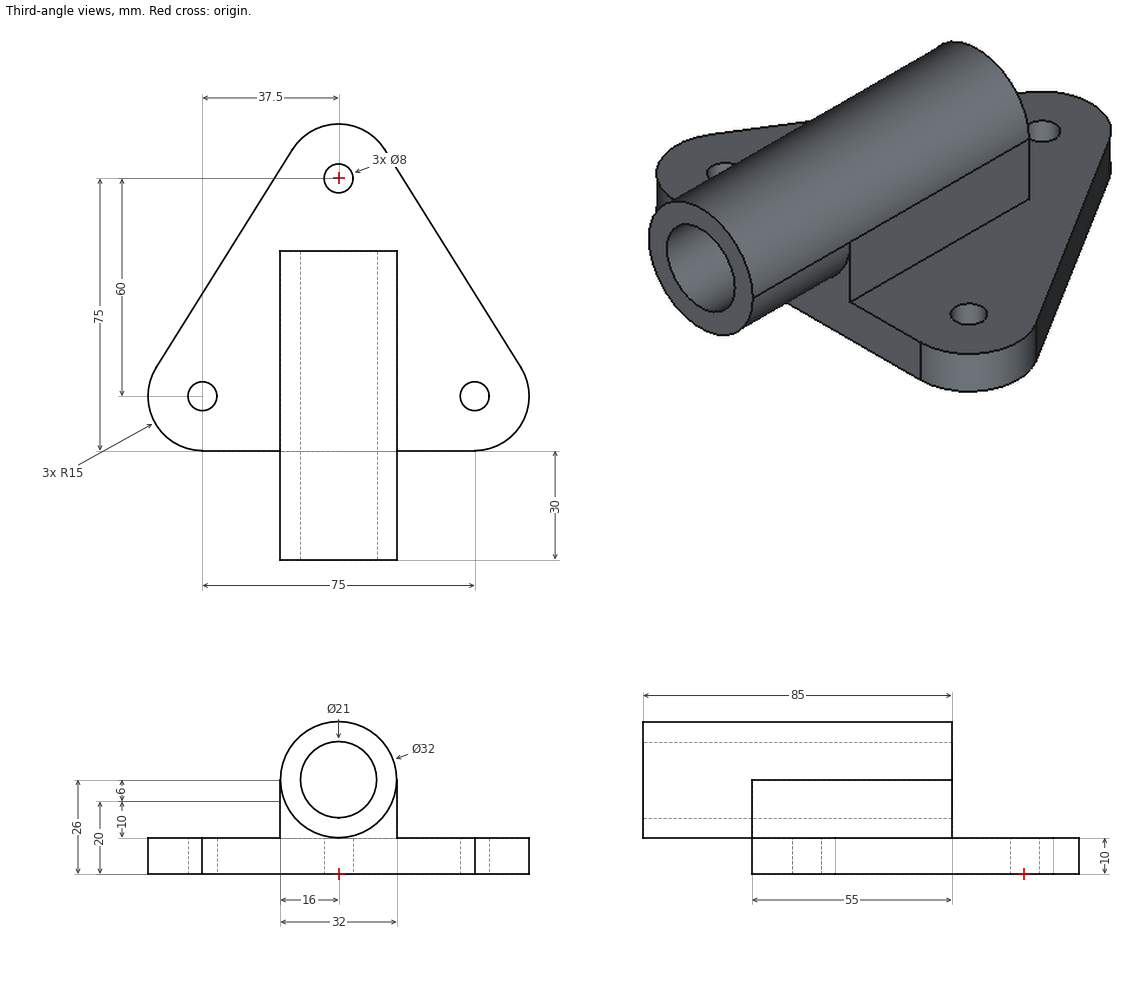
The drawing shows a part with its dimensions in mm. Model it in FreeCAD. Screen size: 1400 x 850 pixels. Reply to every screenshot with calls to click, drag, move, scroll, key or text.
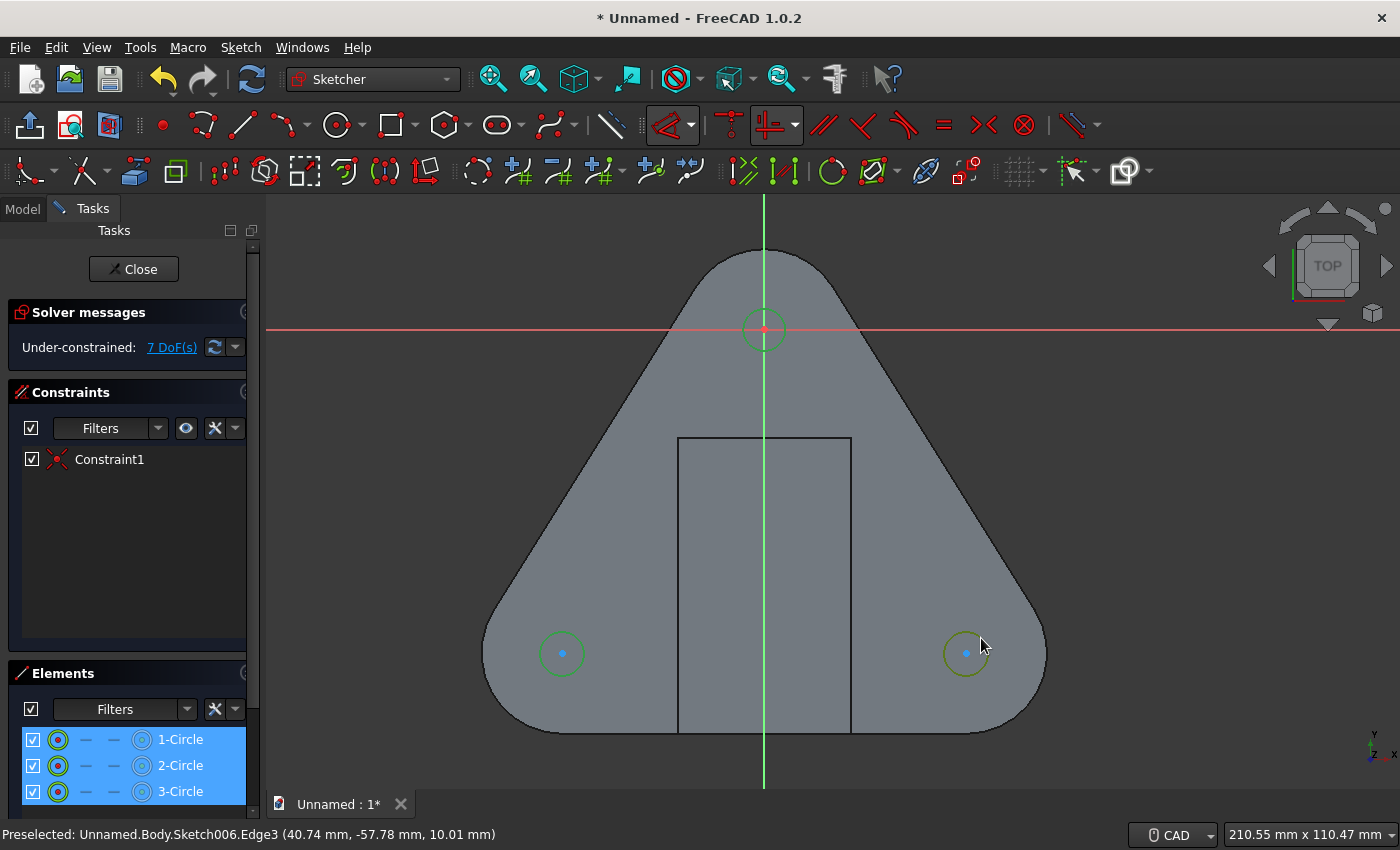
click(944, 126)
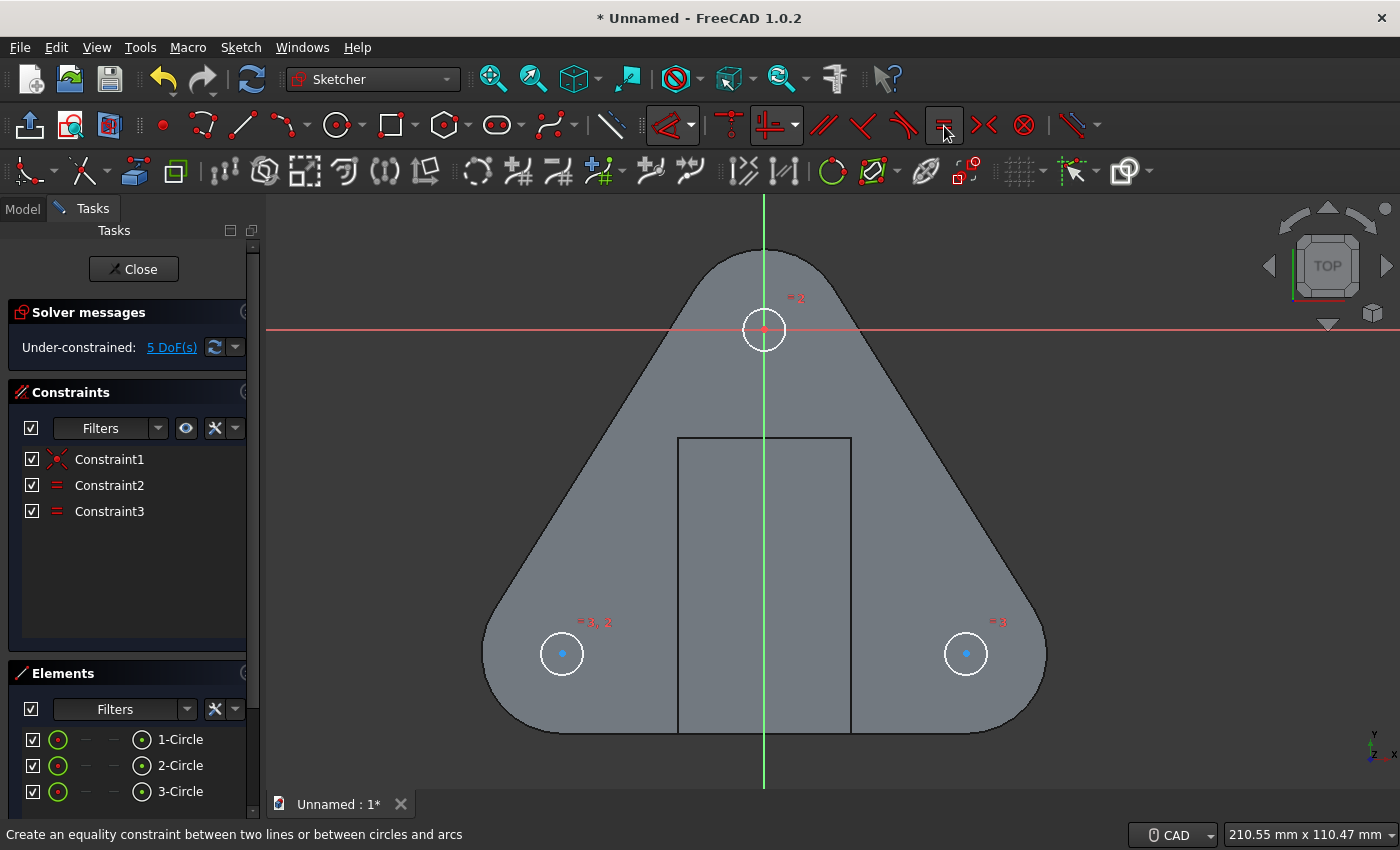
click(562, 654)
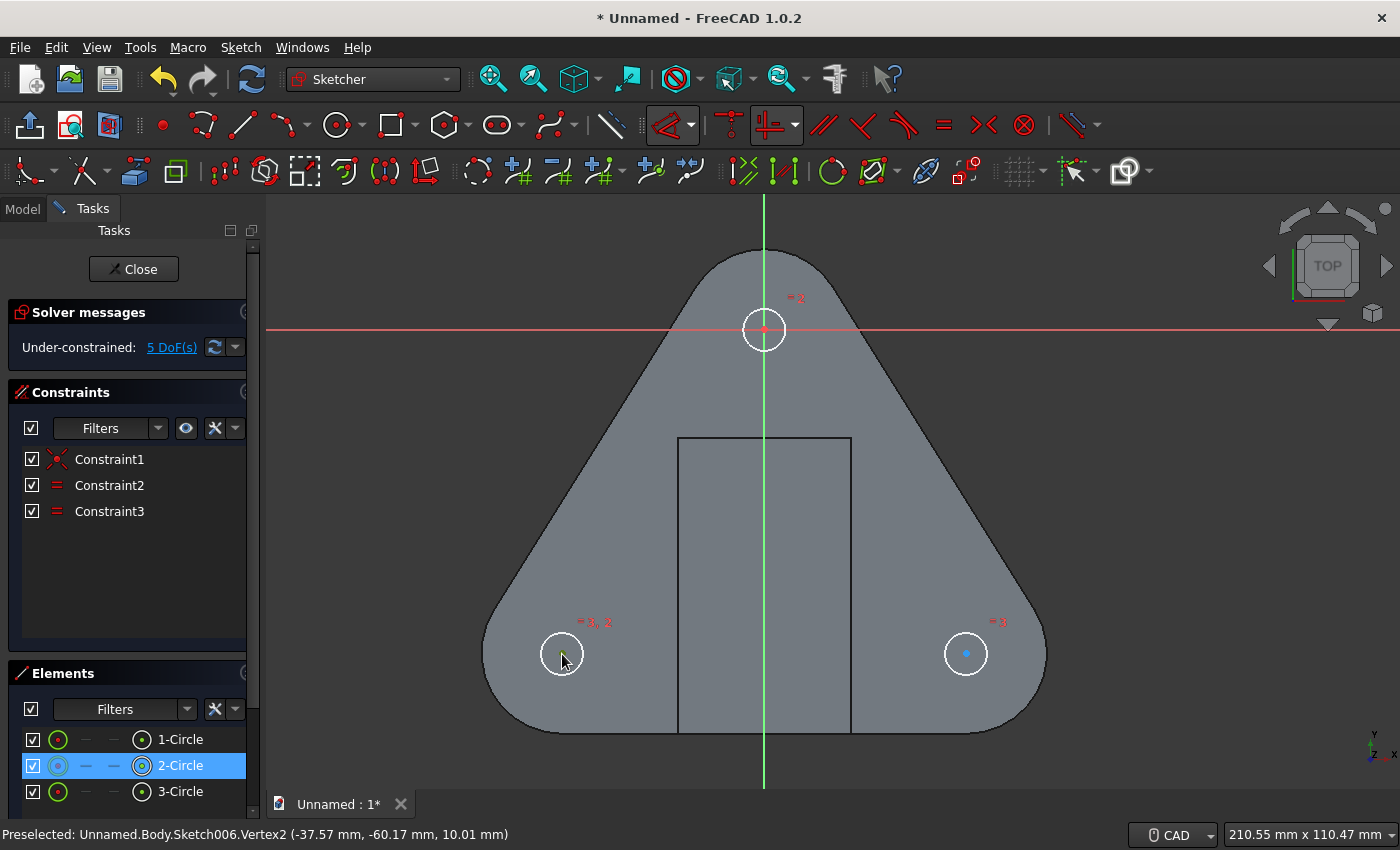
click(966, 654)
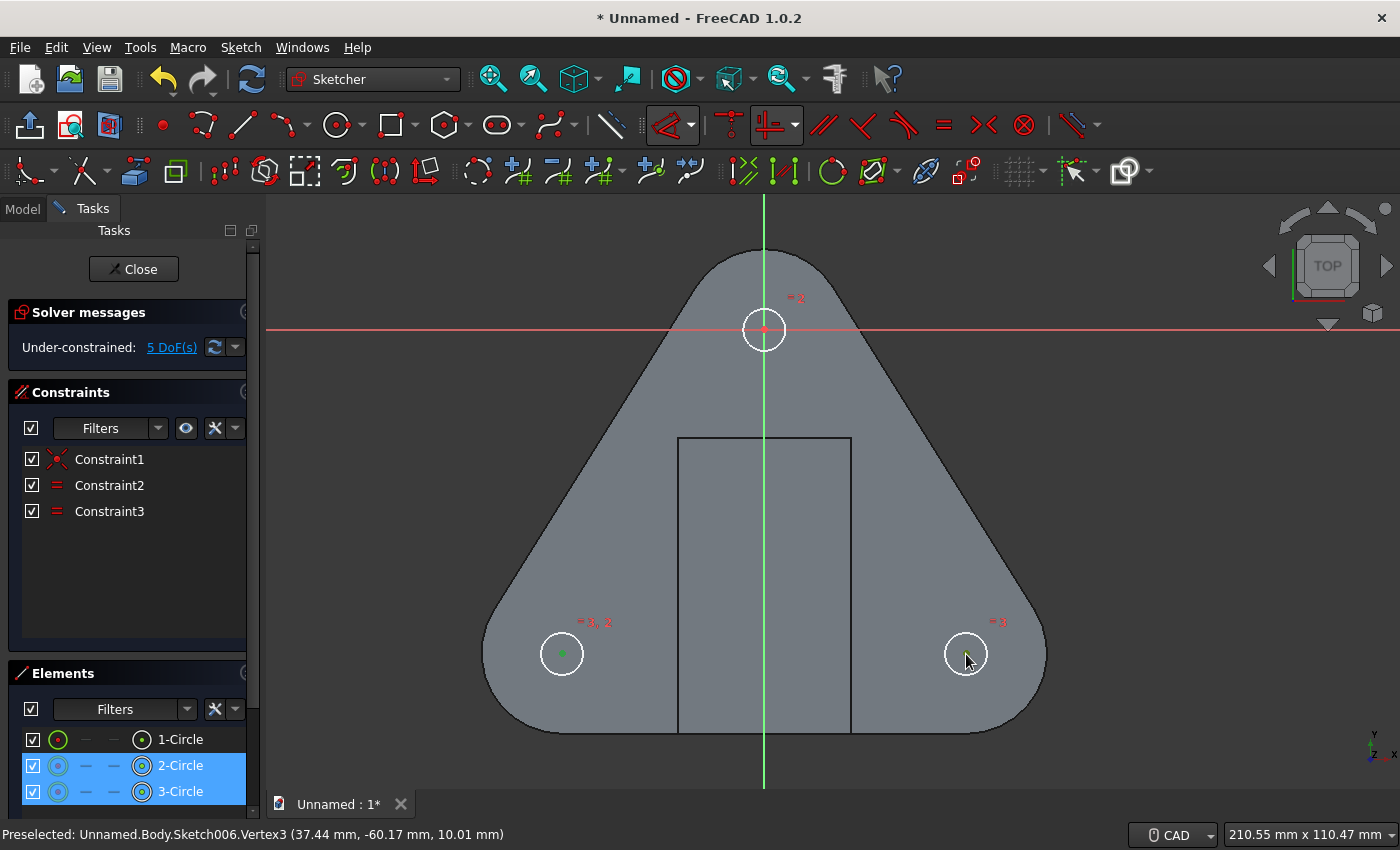
key(h)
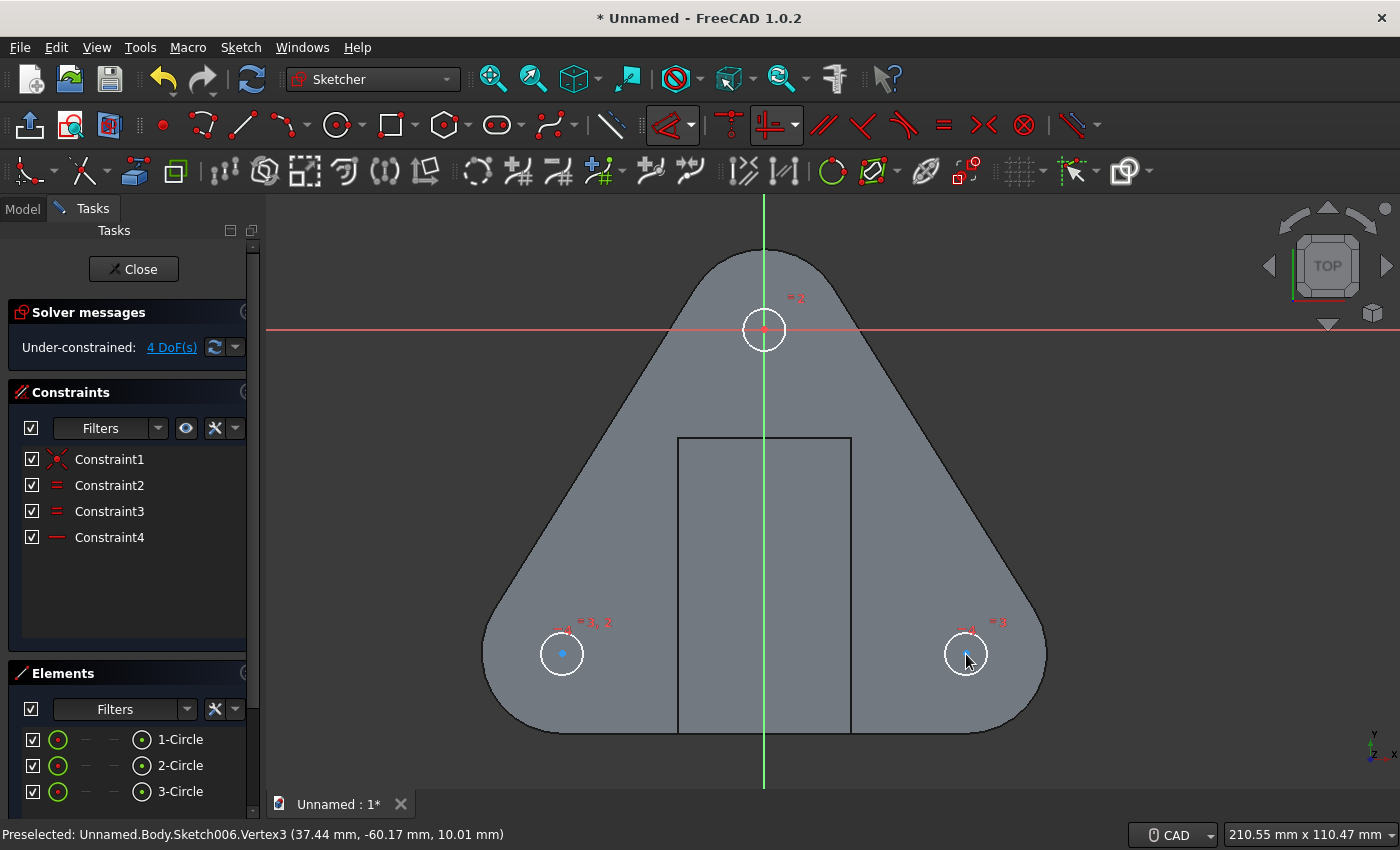
click(779, 315)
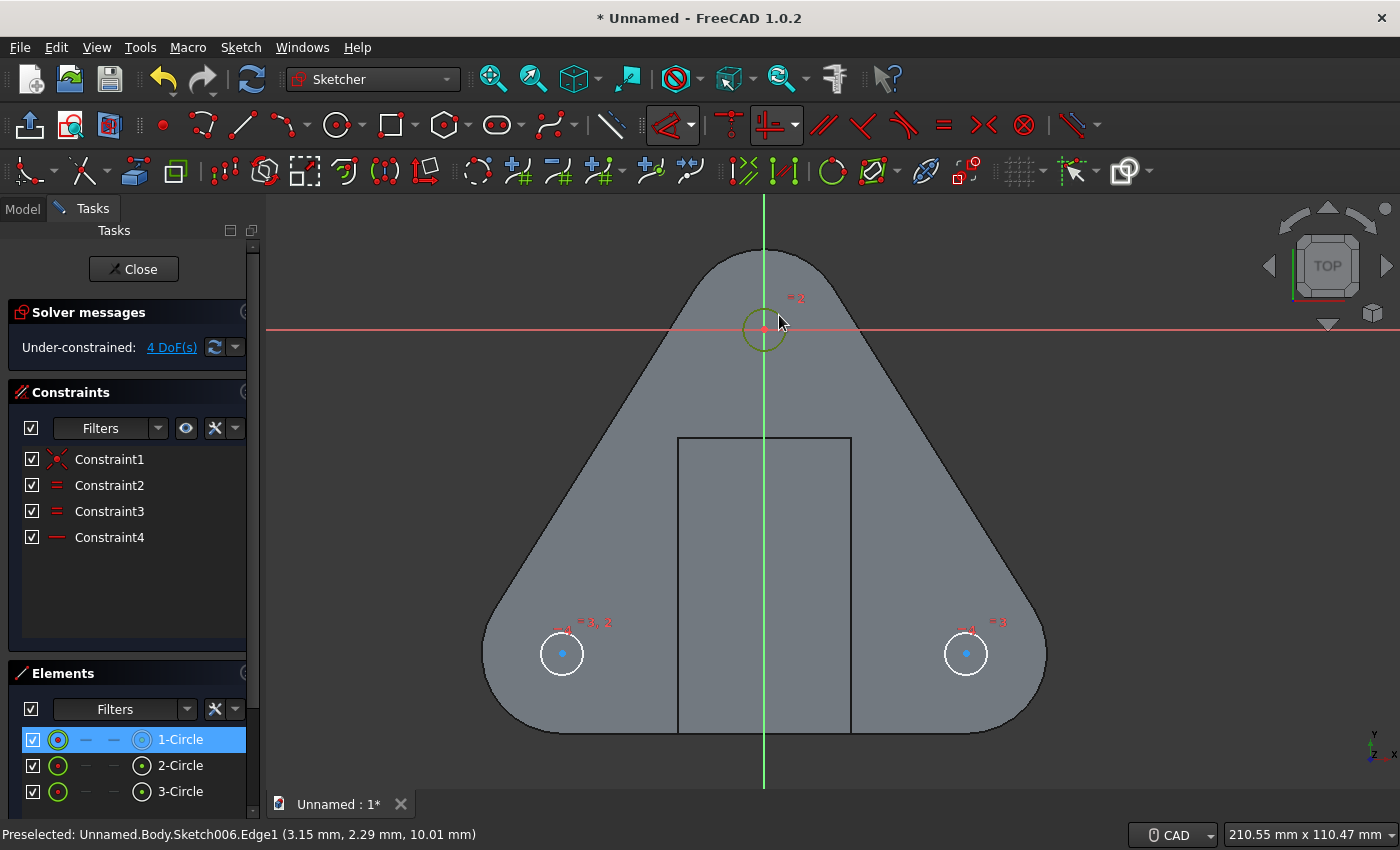
click(694, 126)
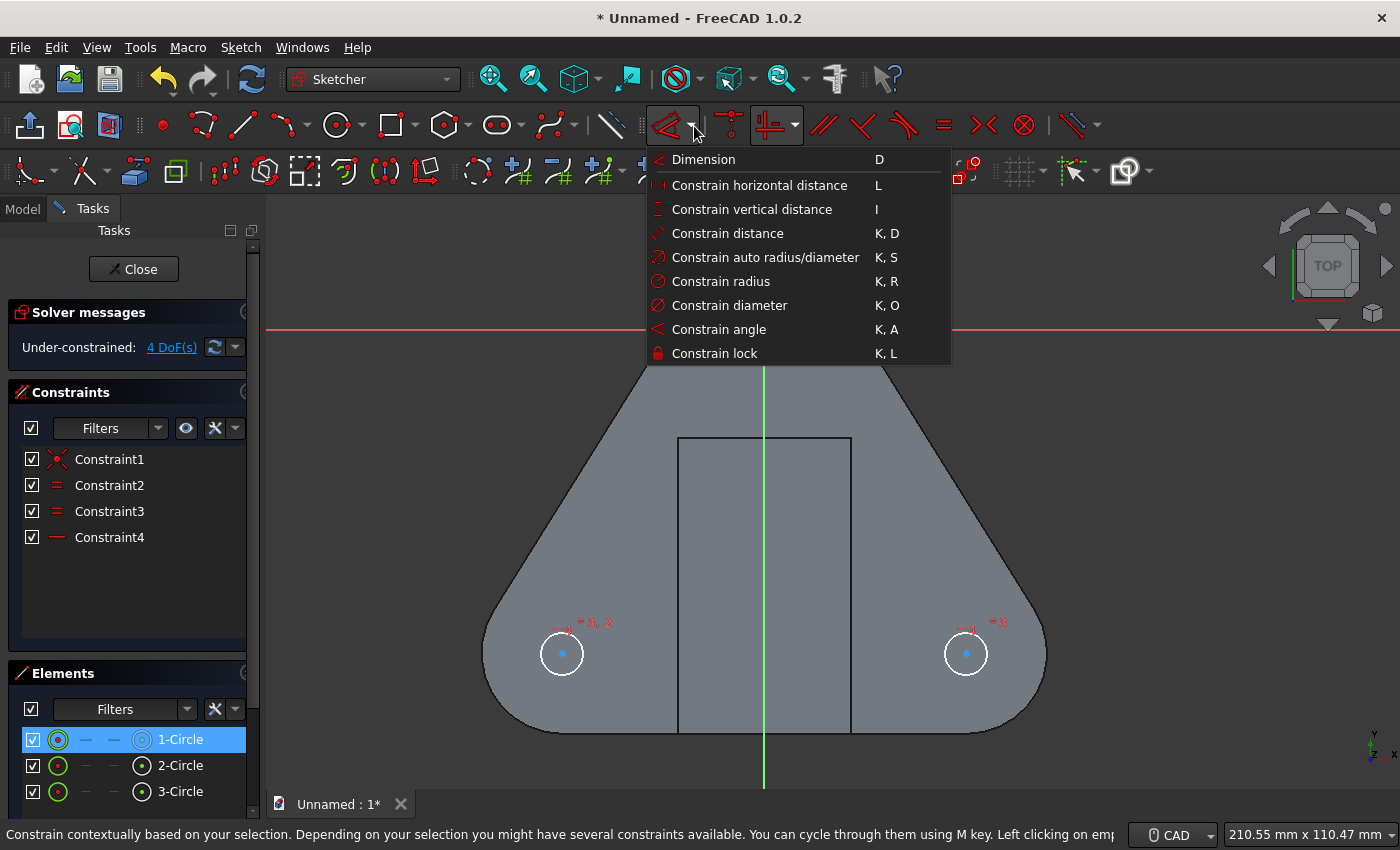
click(799, 305)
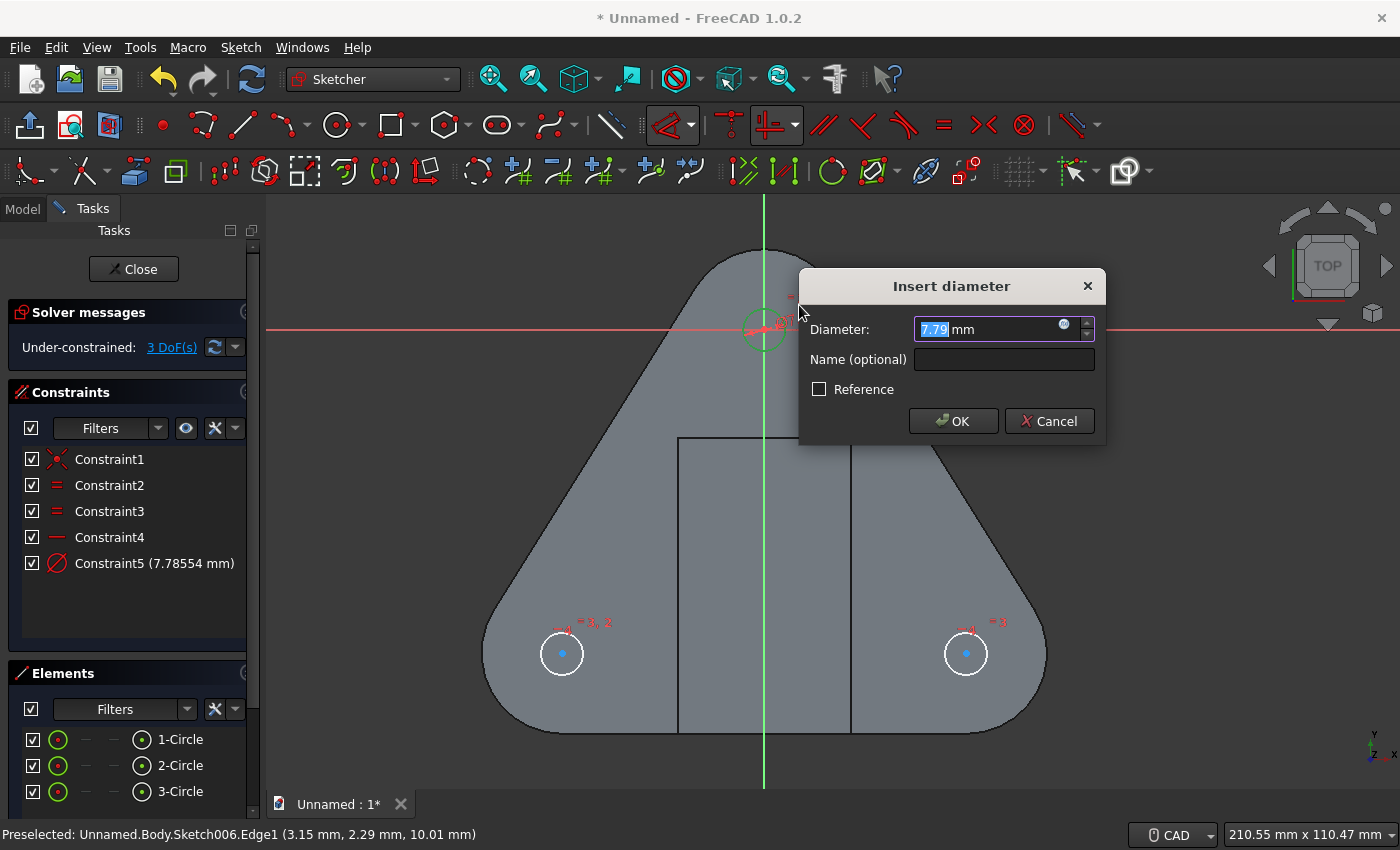
text(8)
key(Return)